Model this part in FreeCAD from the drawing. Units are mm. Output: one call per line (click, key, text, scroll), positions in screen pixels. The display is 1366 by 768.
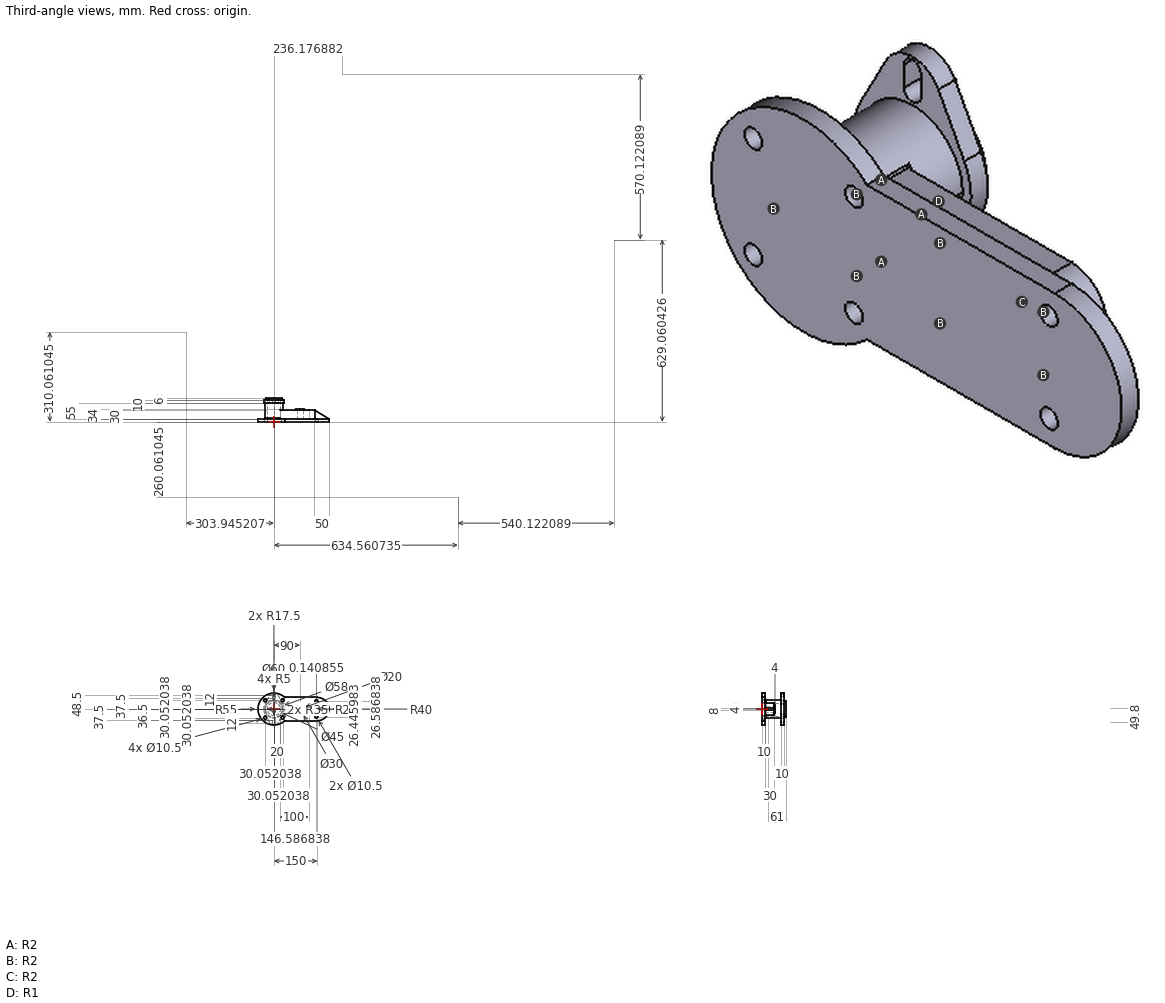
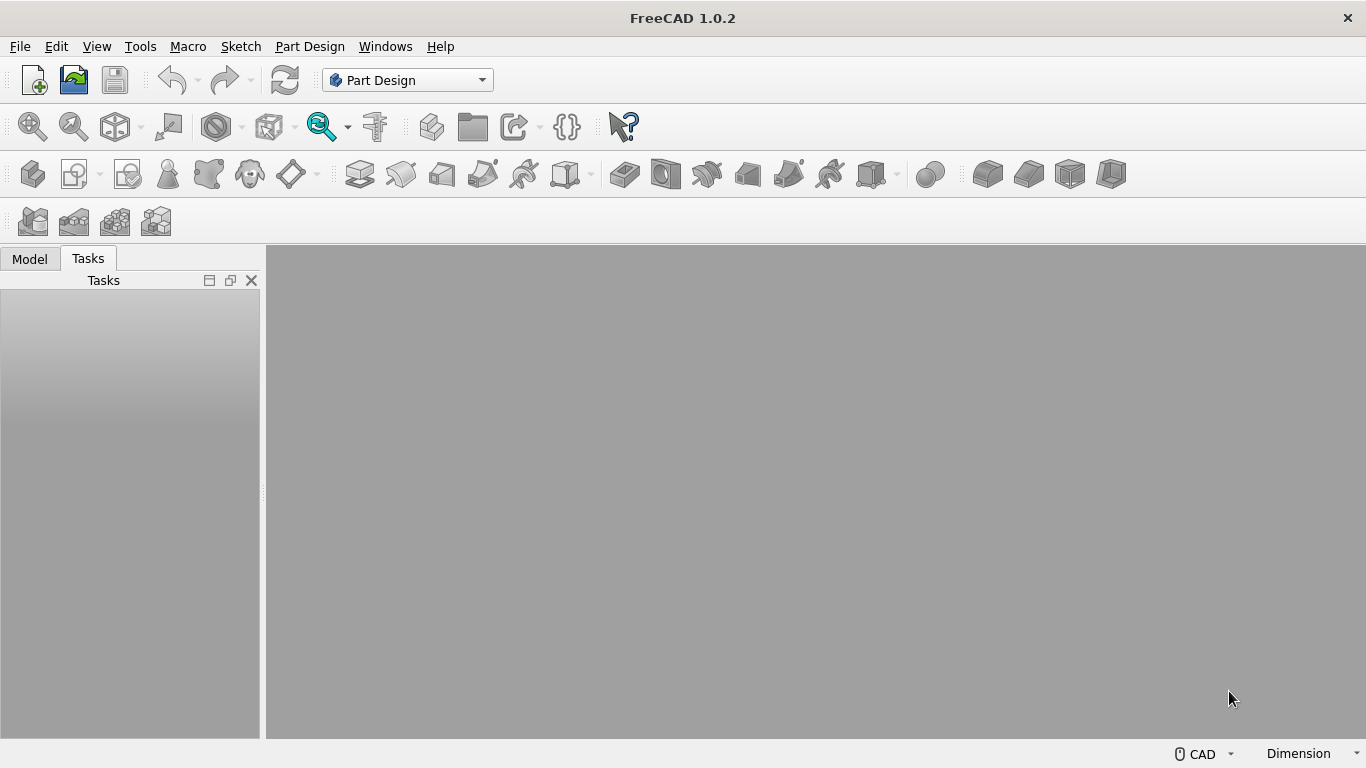
click(33, 80)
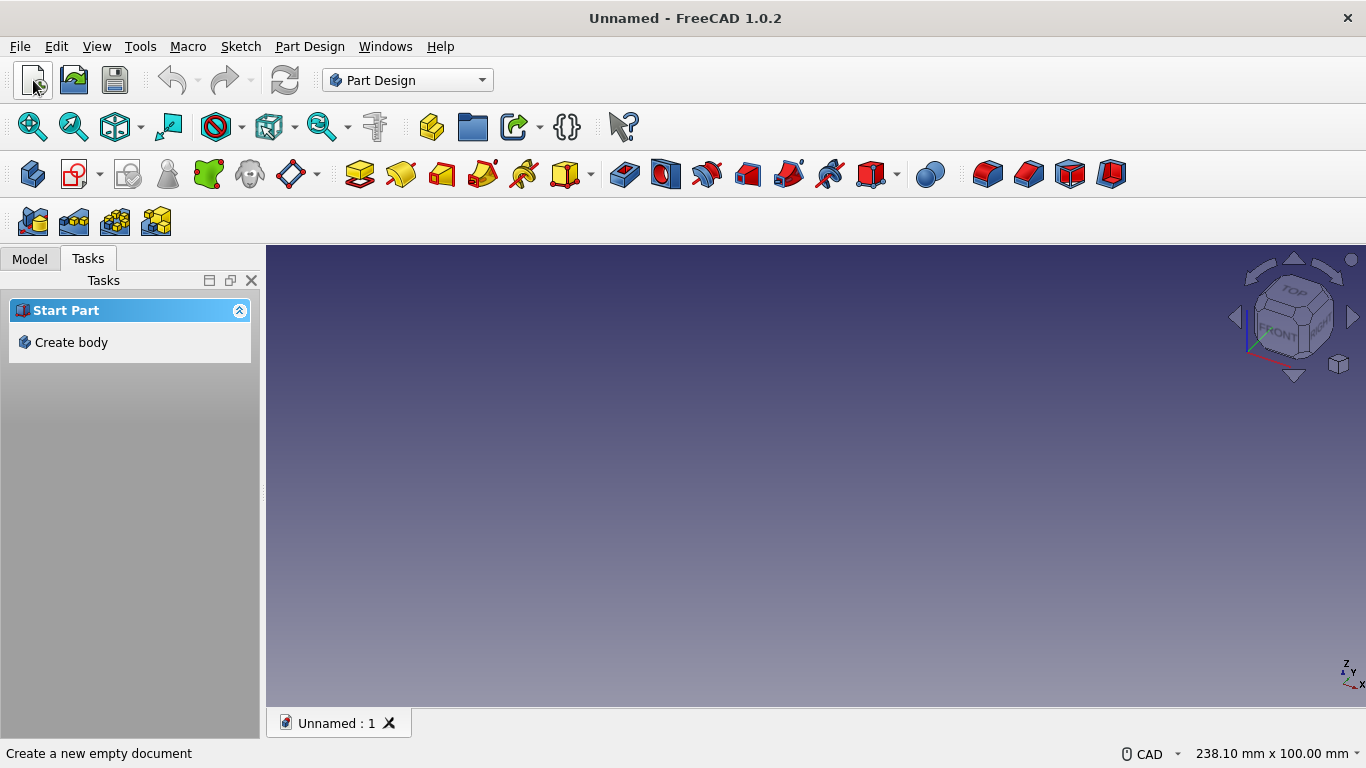
click(74, 174)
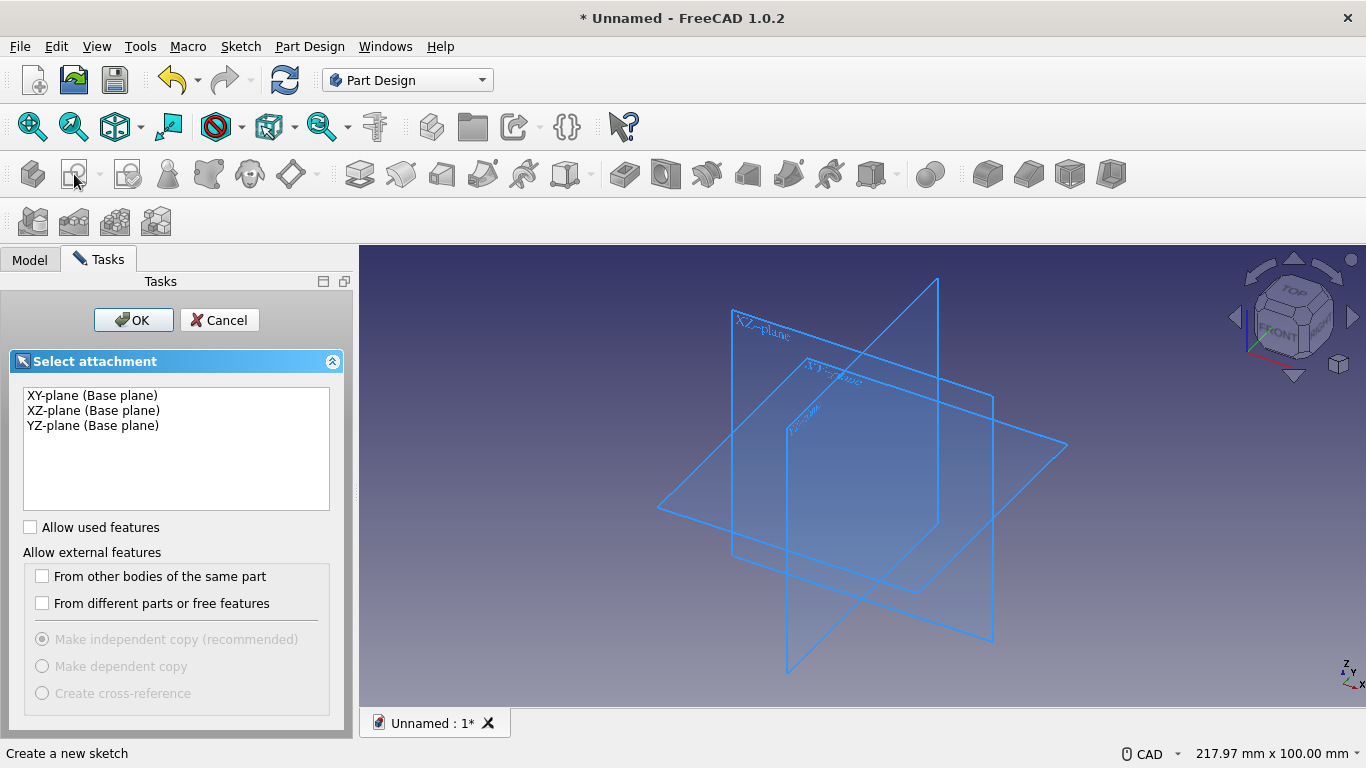
click(84, 410)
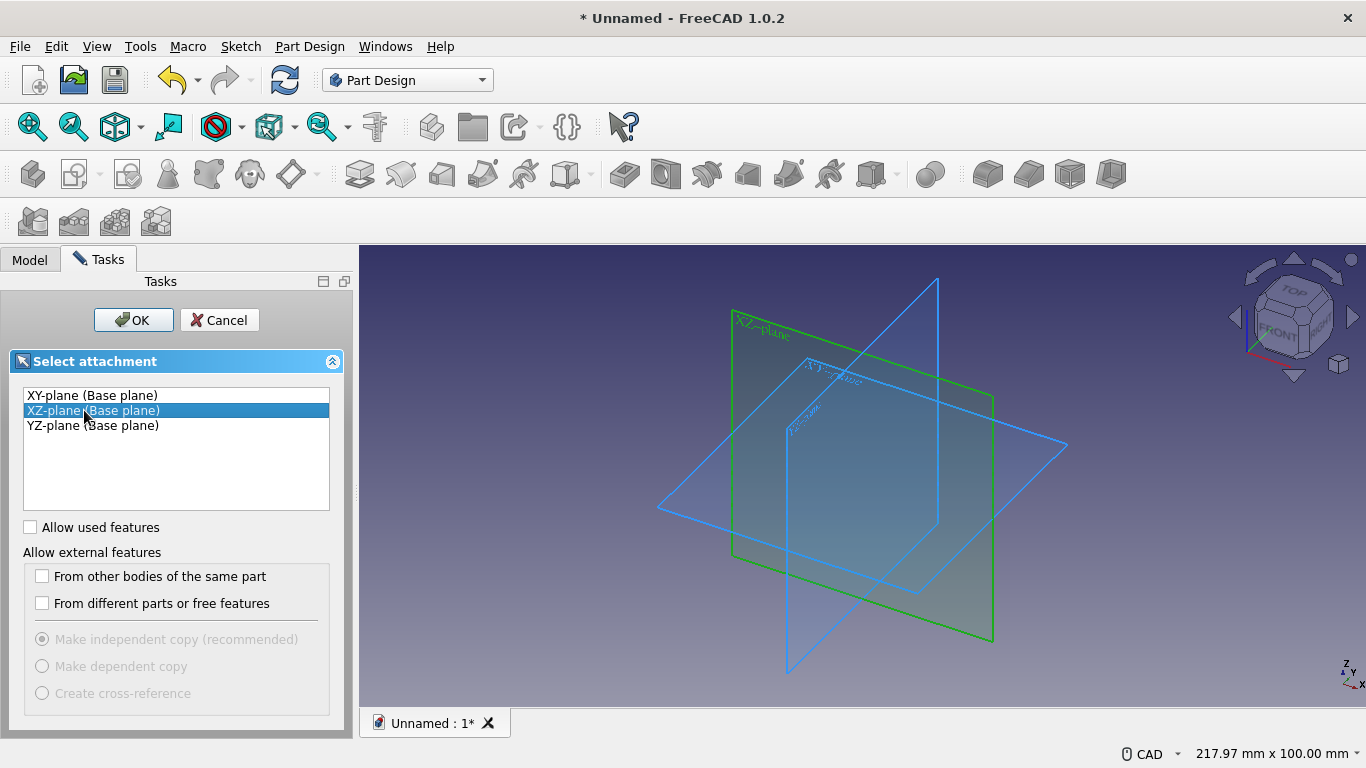
click(134, 320)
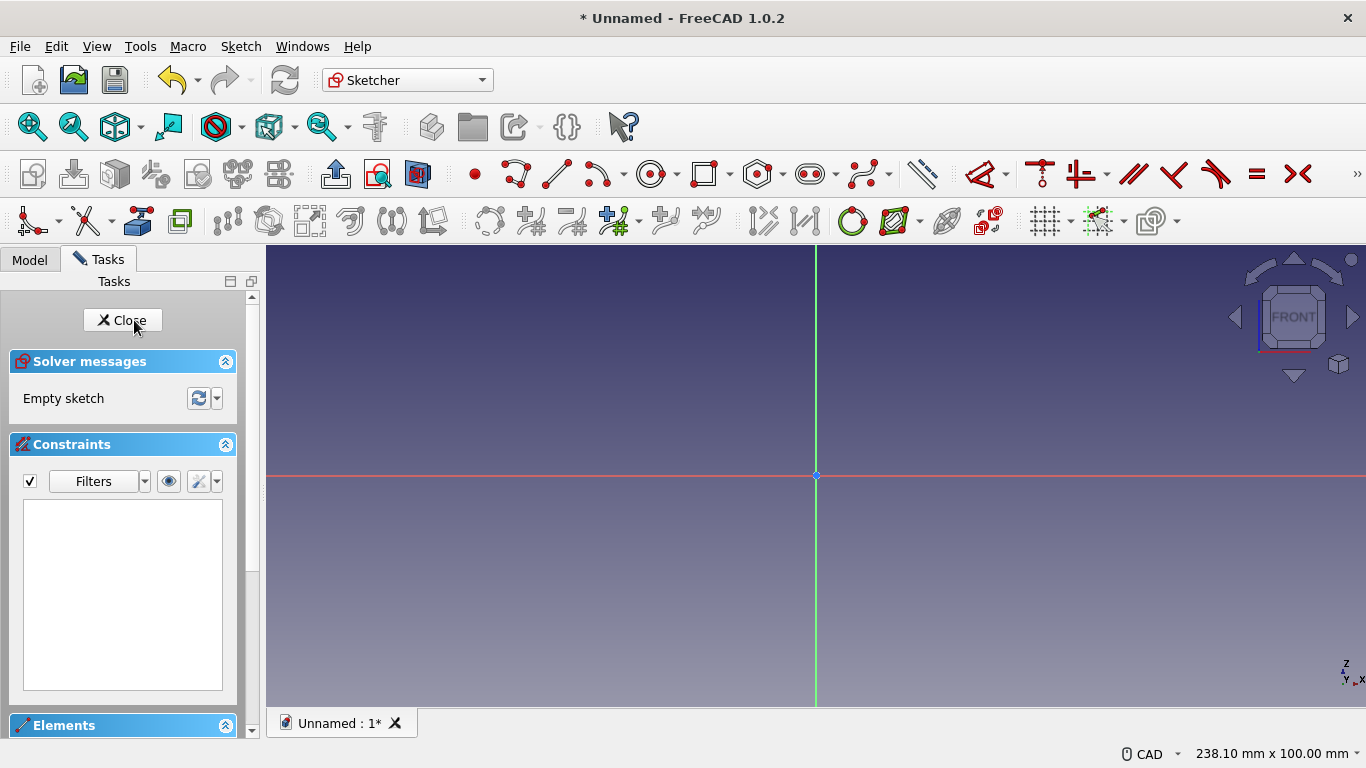
scroll(294, 476, down, 3)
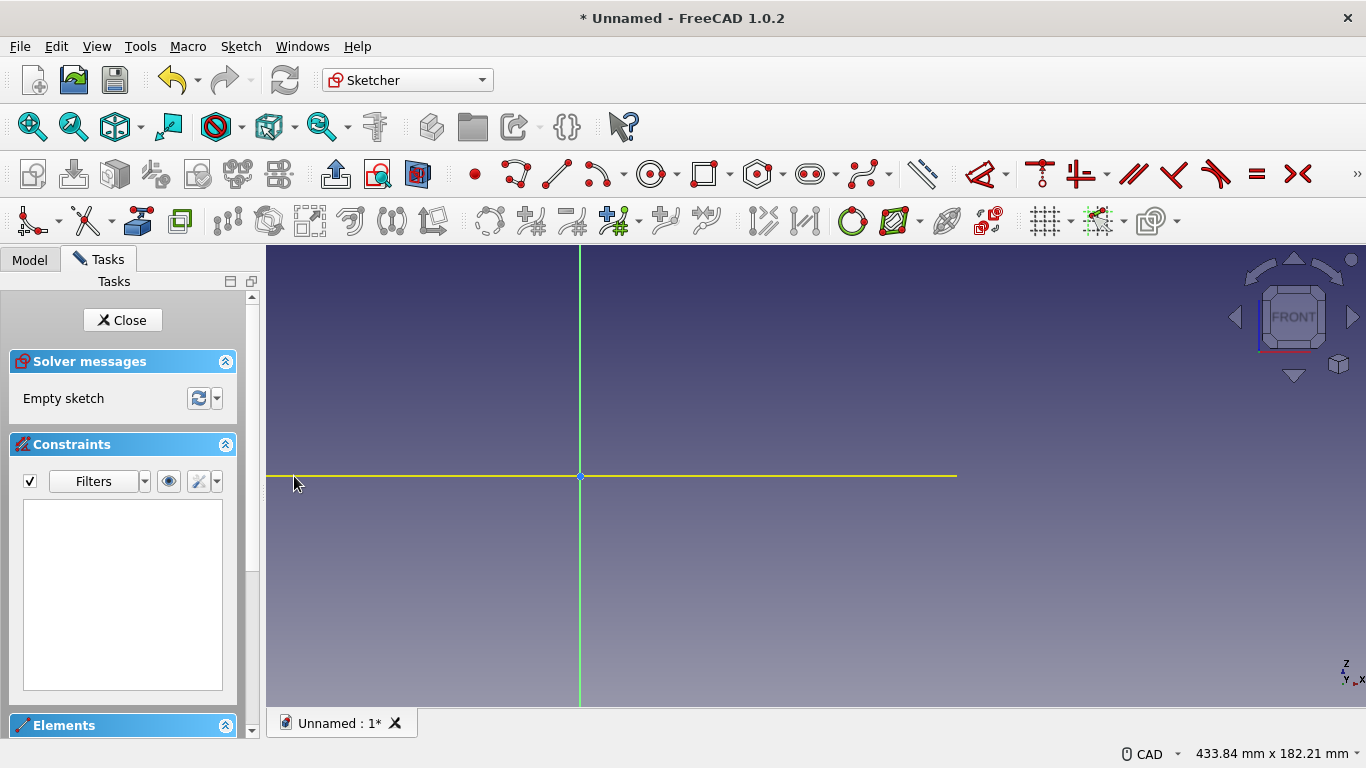
click(557, 174)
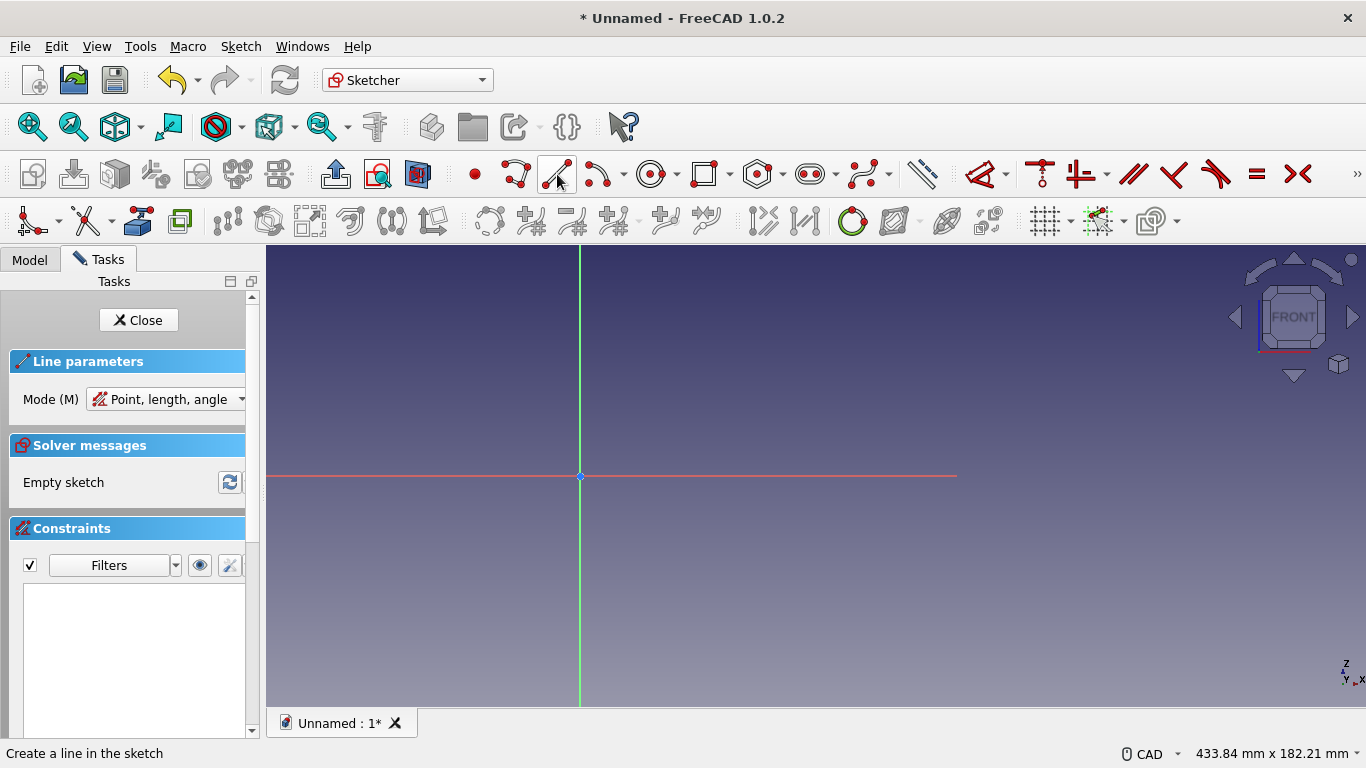
click(961, 578)
click(676, 578)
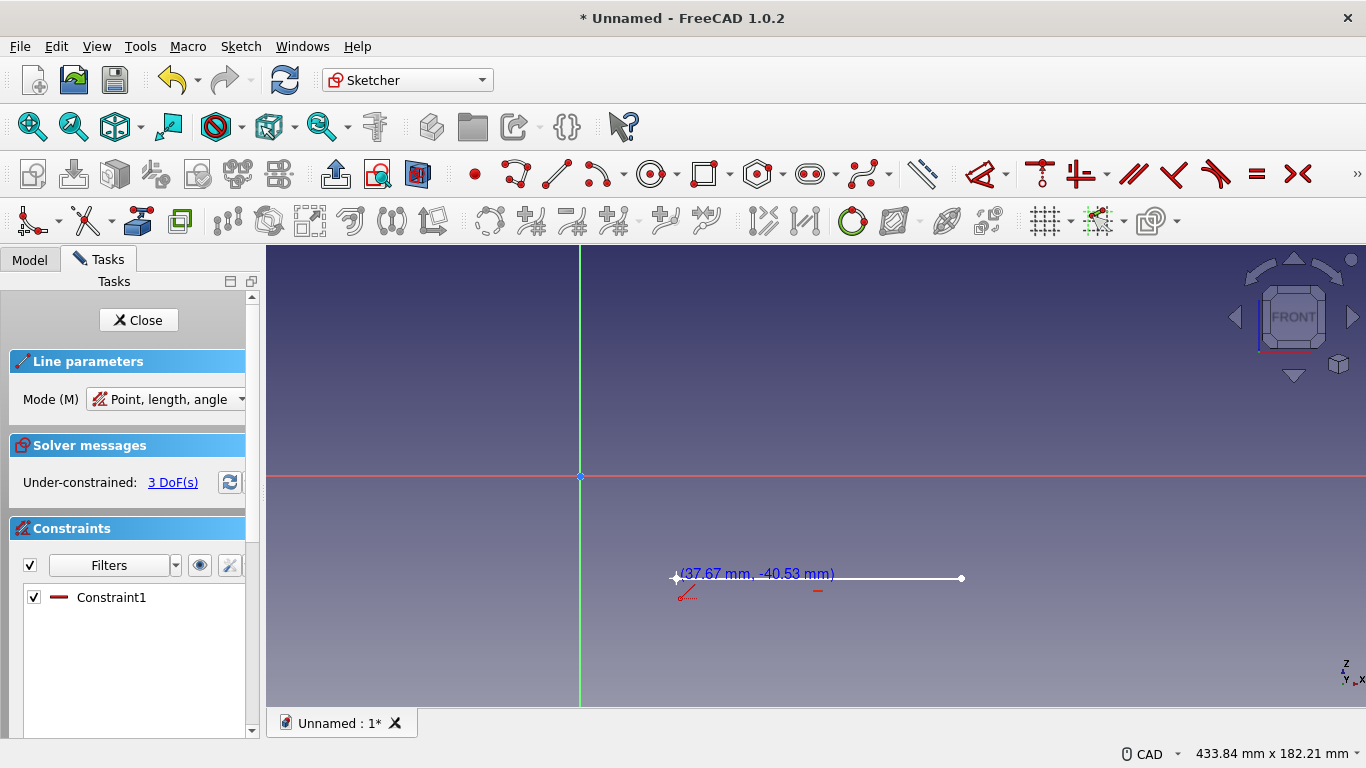
click(676, 375)
click(961, 375)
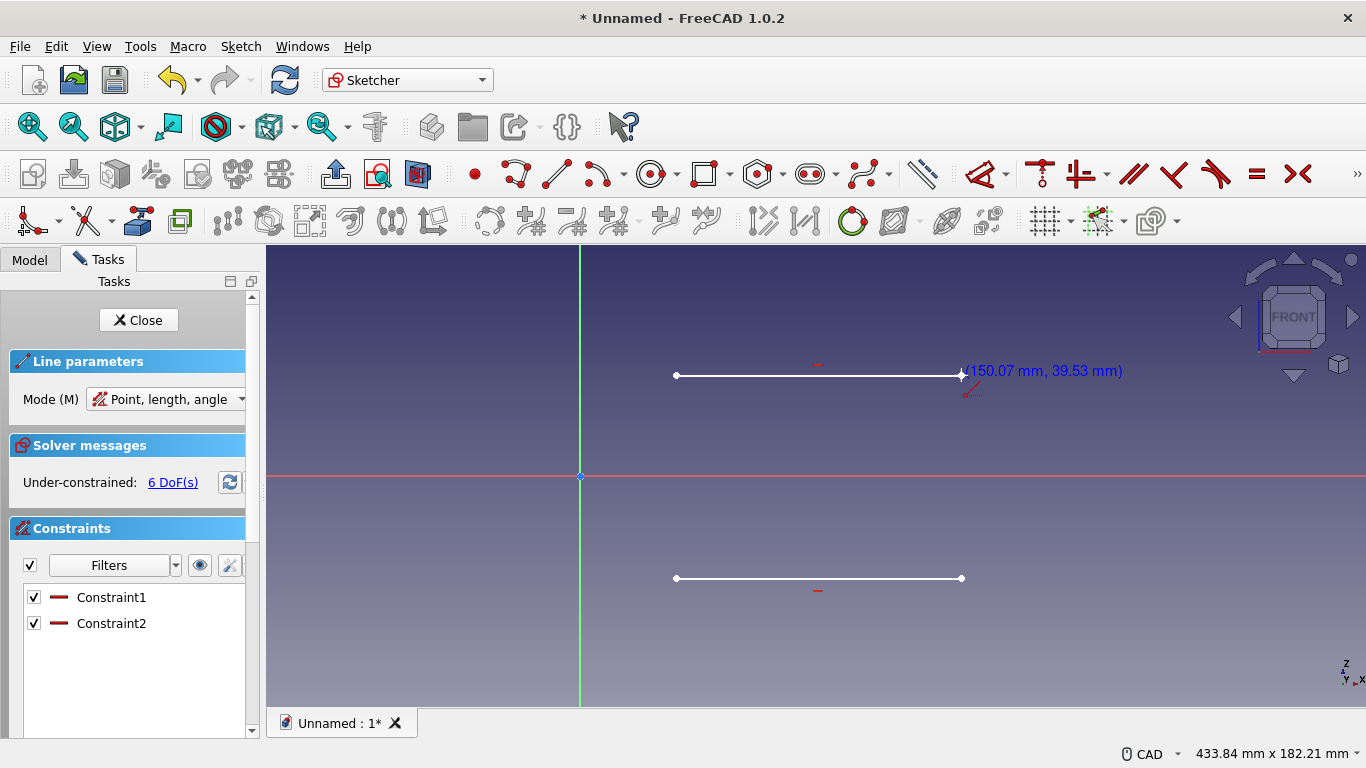
key(g)
key(3)
key(a)